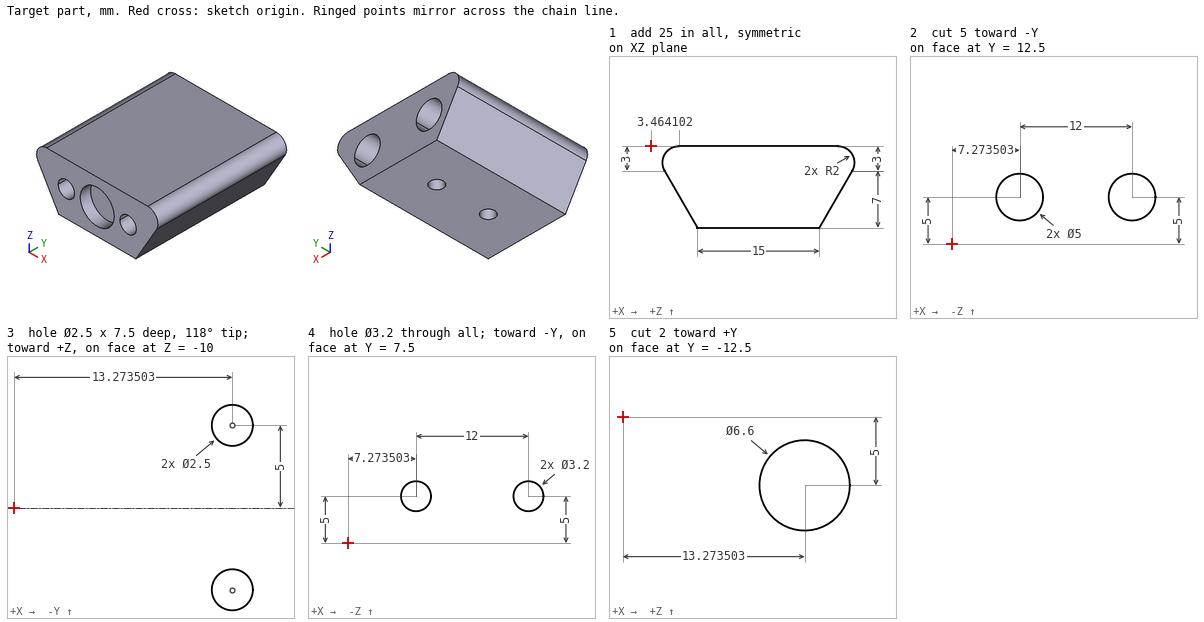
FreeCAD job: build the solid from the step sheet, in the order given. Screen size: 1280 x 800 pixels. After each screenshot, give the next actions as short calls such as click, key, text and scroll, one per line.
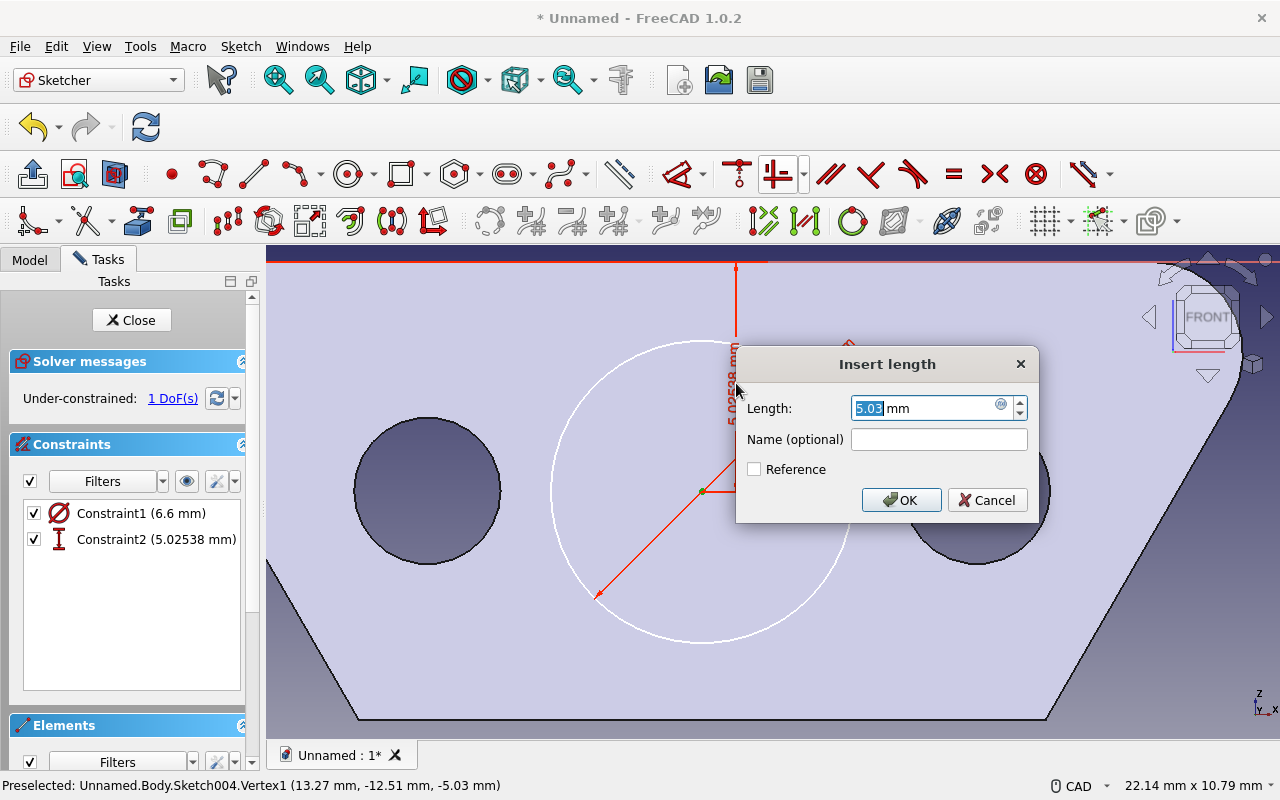
text(5)
key(Return)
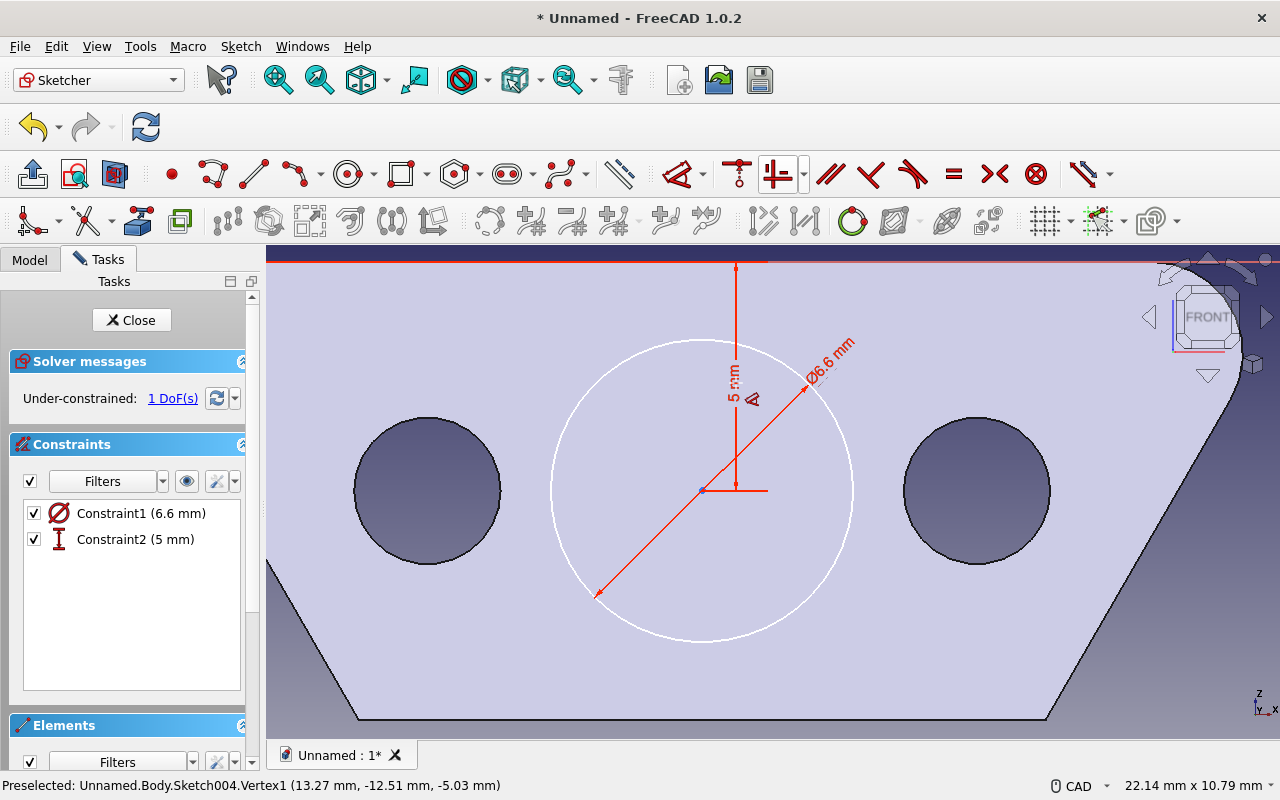
click(702, 491)
click(498, 525)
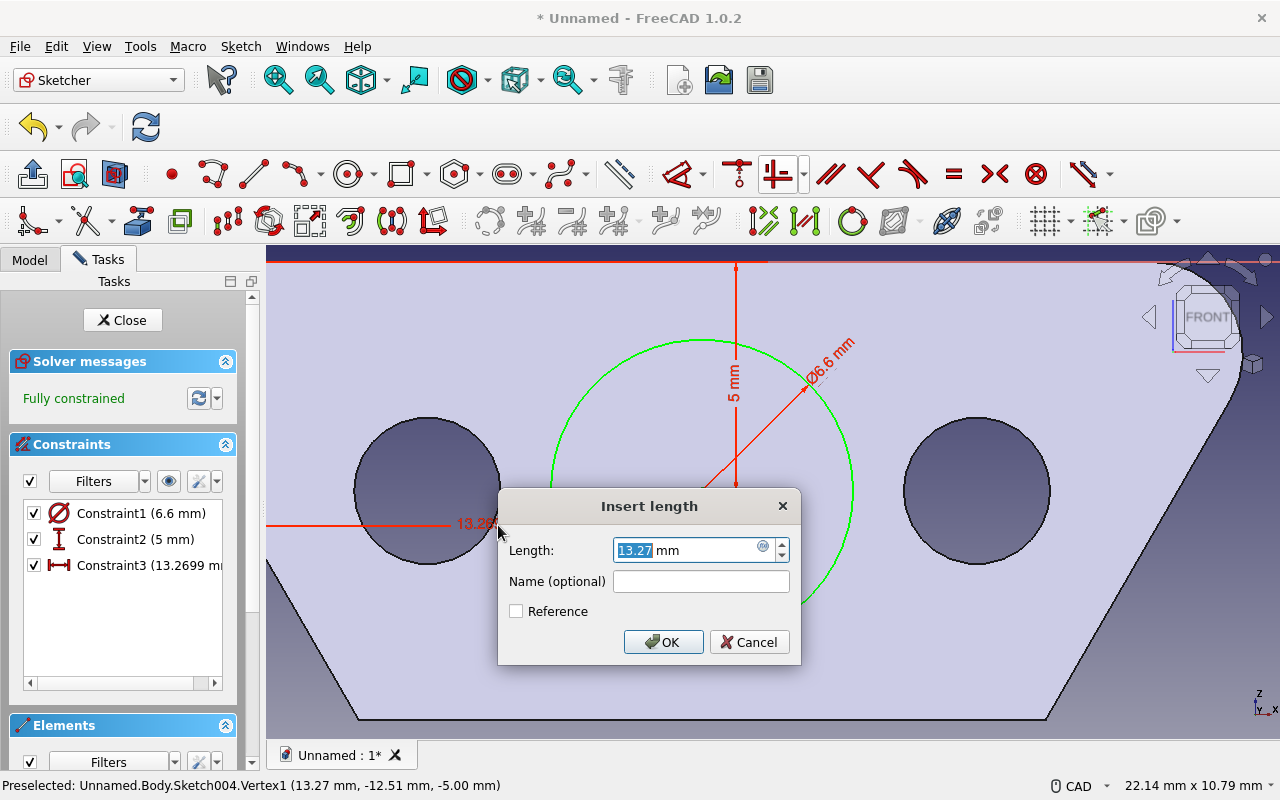
text(13.273503)
key(Return)
key(Escape)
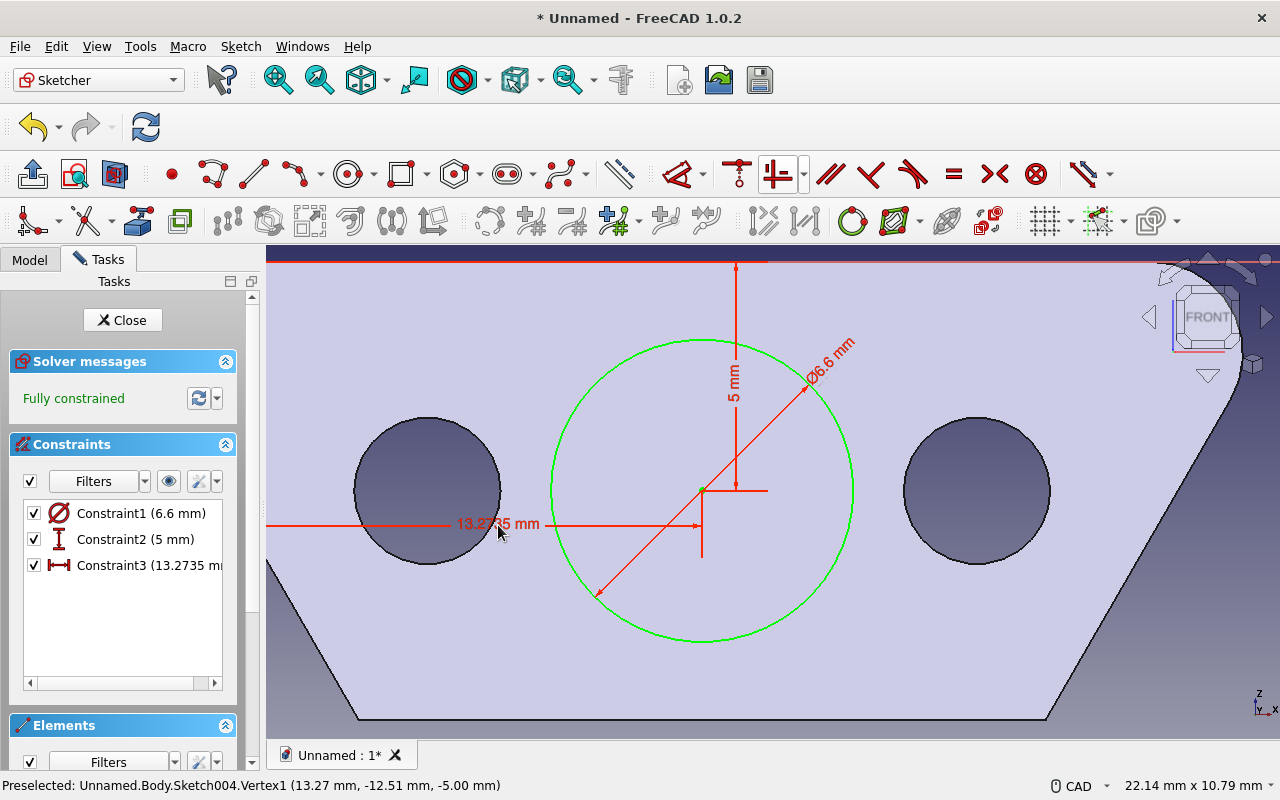
click(123, 320)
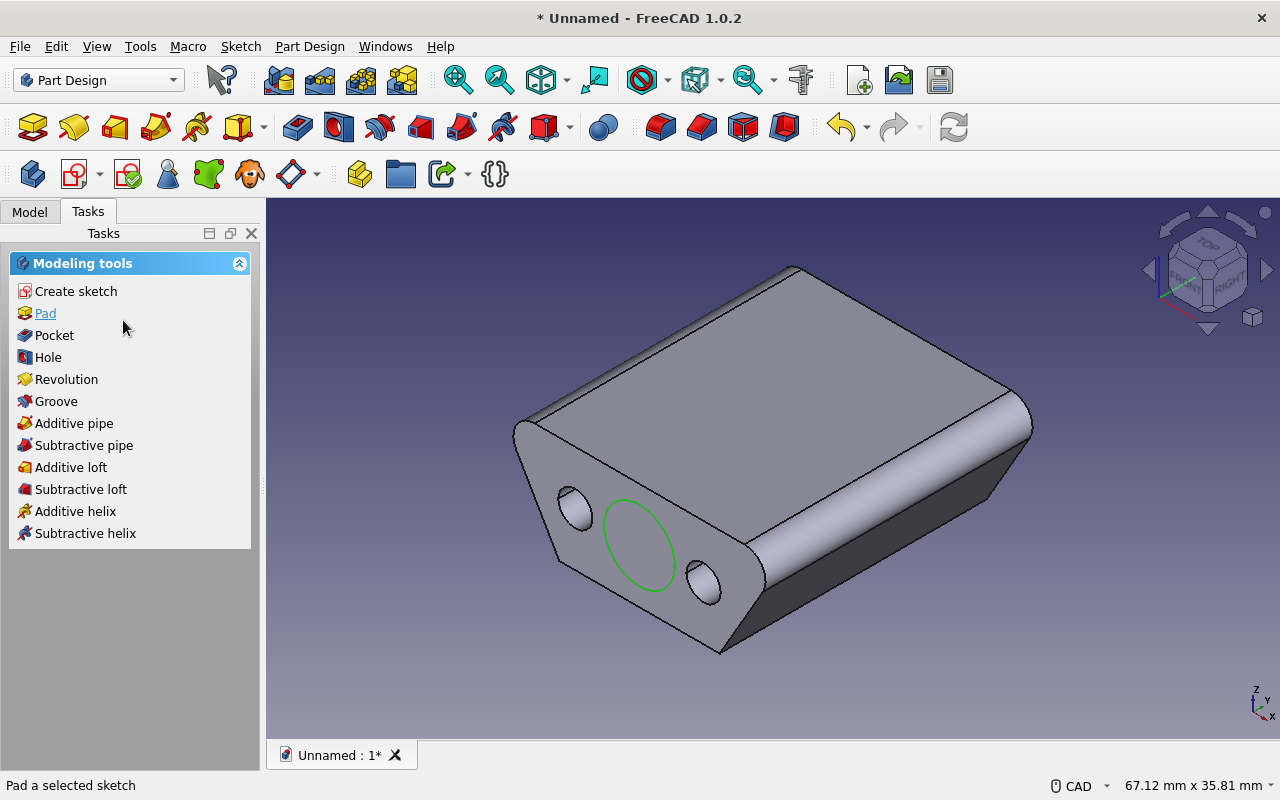
click(298, 128)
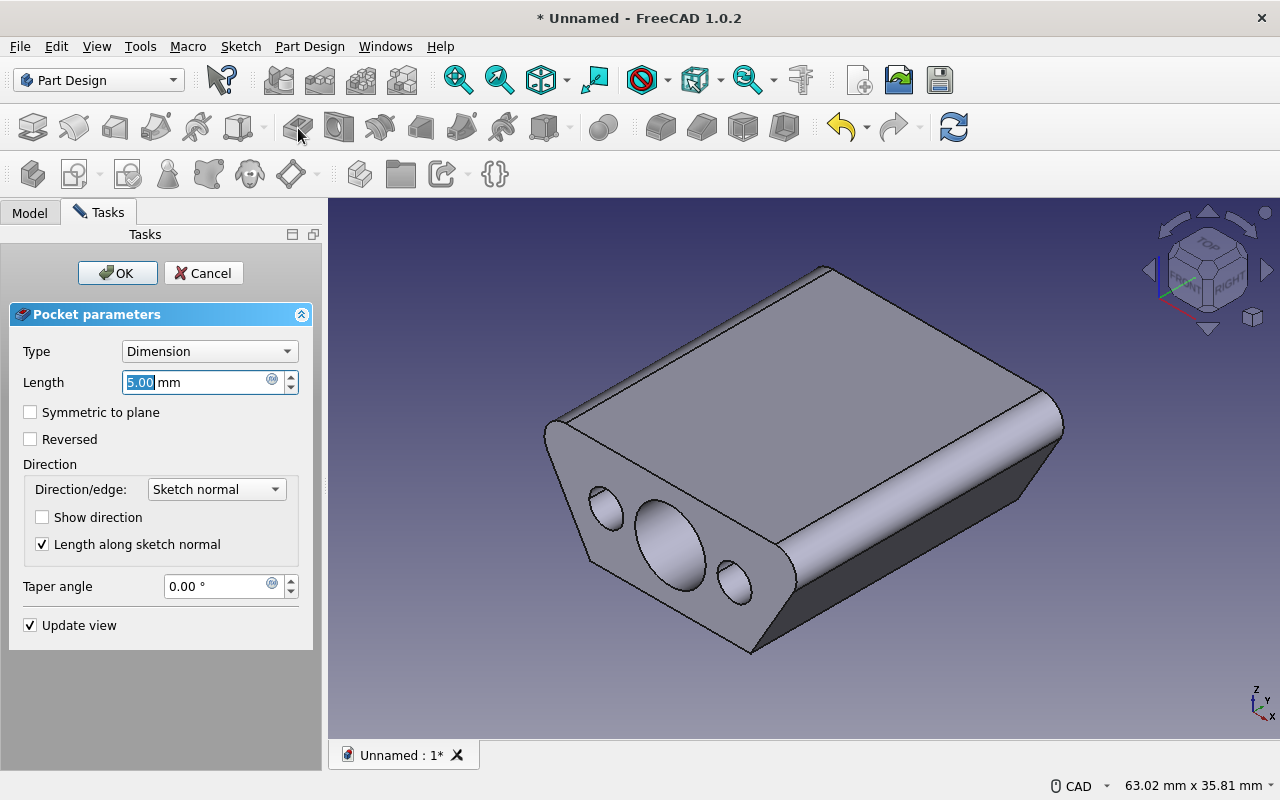
text(2)
key(Tab)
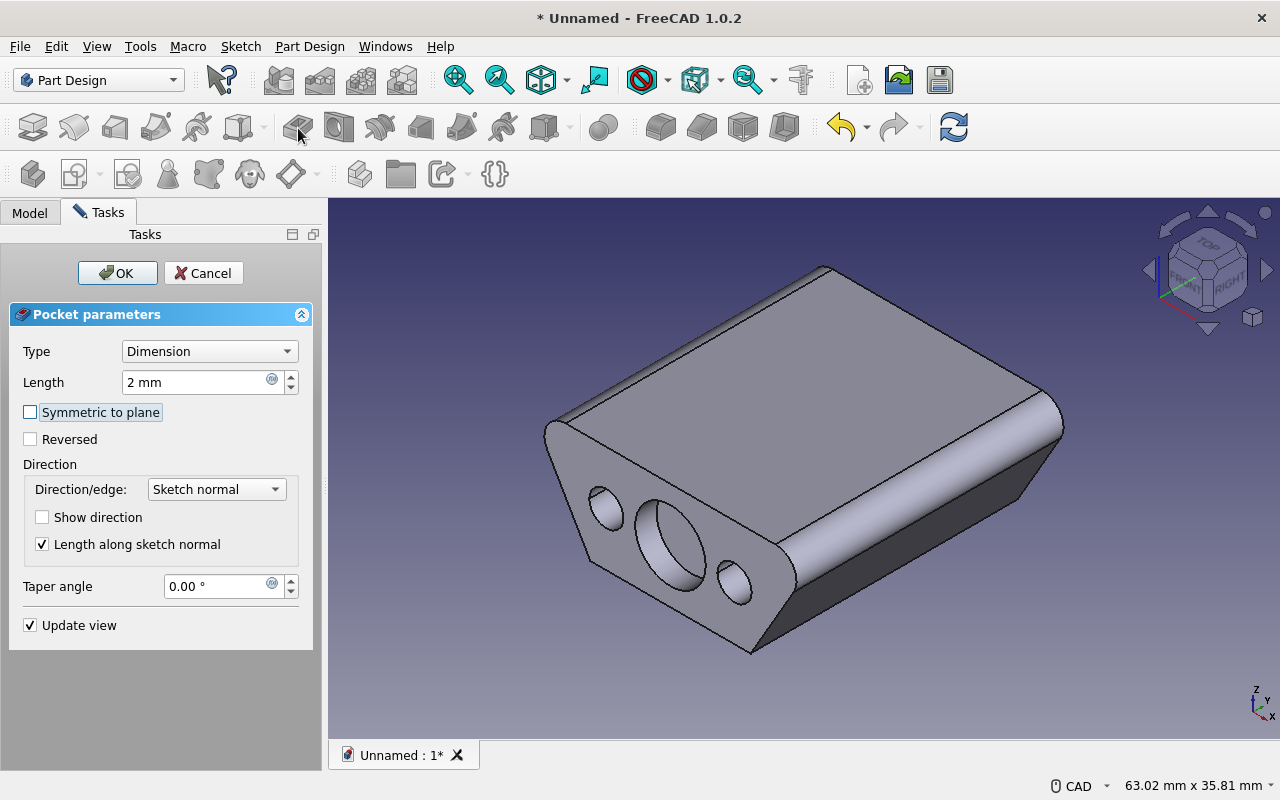
click(118, 273)